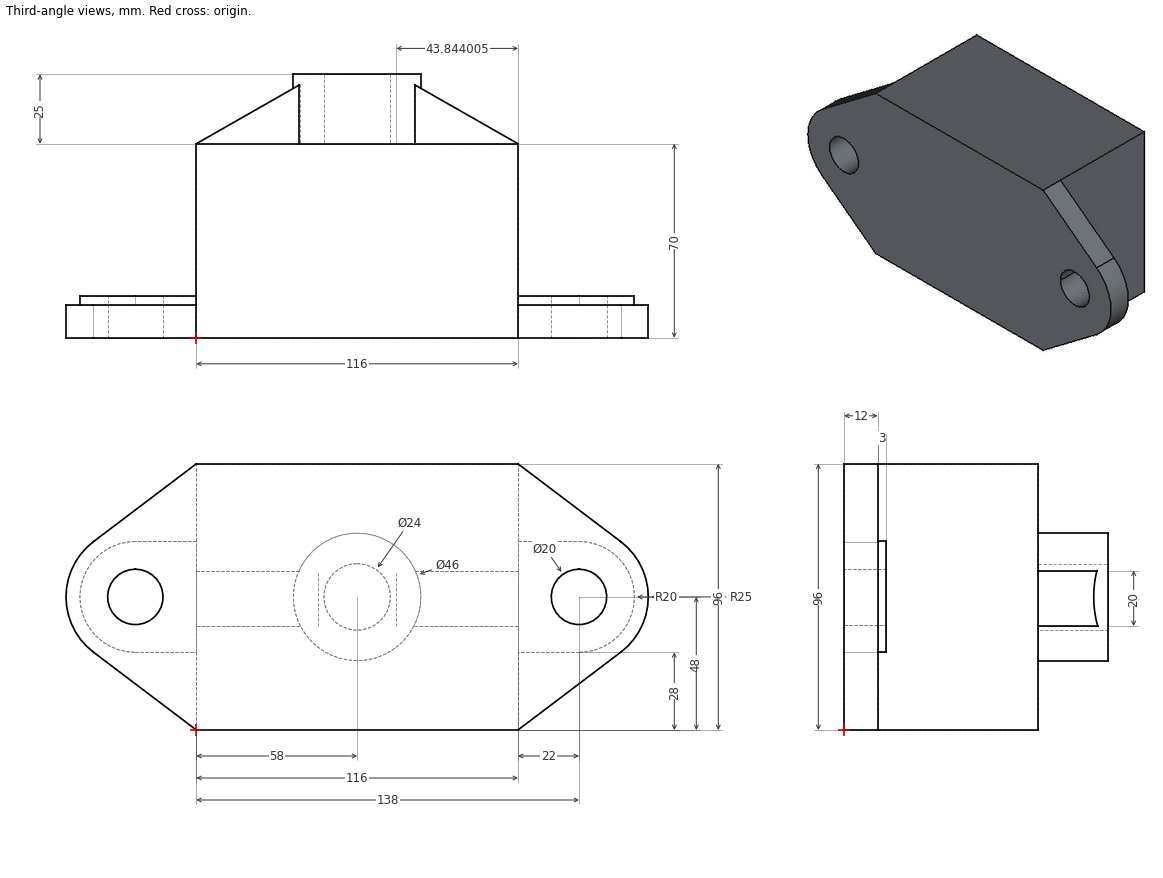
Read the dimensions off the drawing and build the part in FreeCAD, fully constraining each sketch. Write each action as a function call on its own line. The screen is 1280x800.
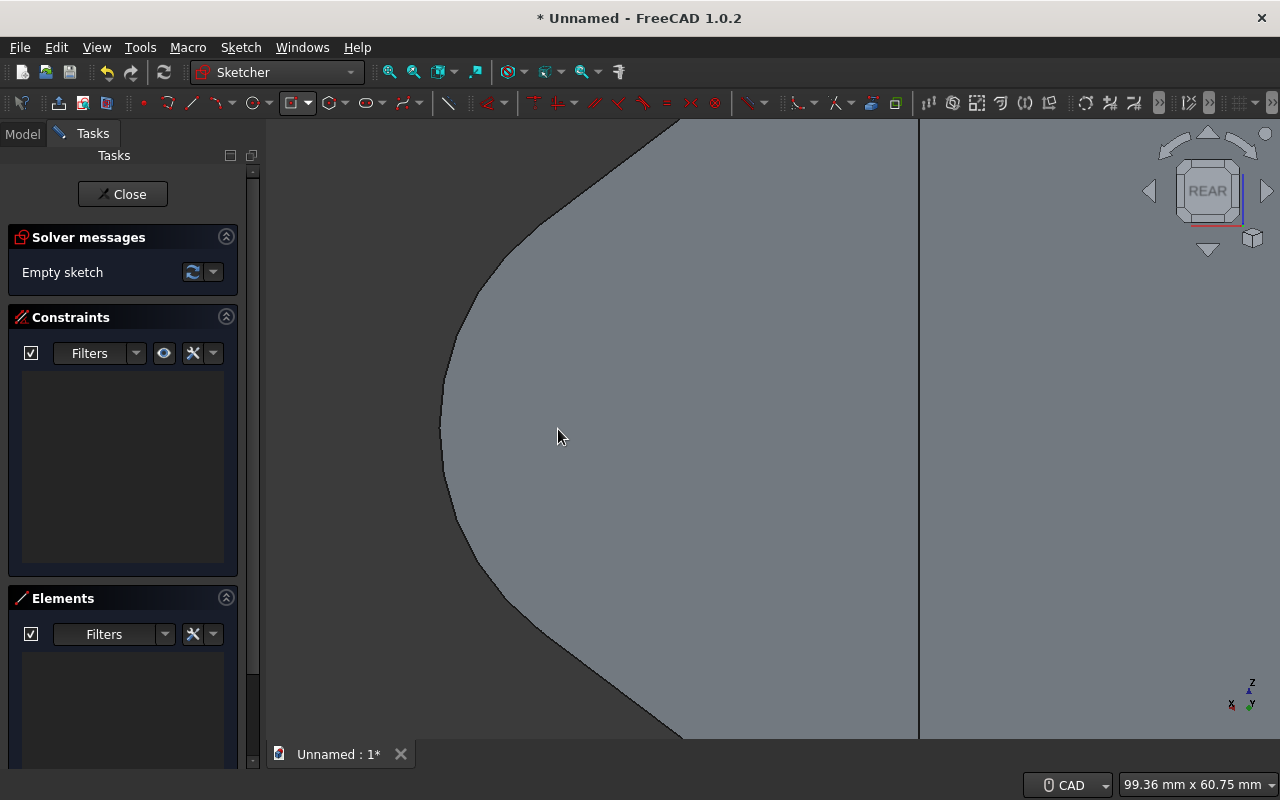
click(168, 104)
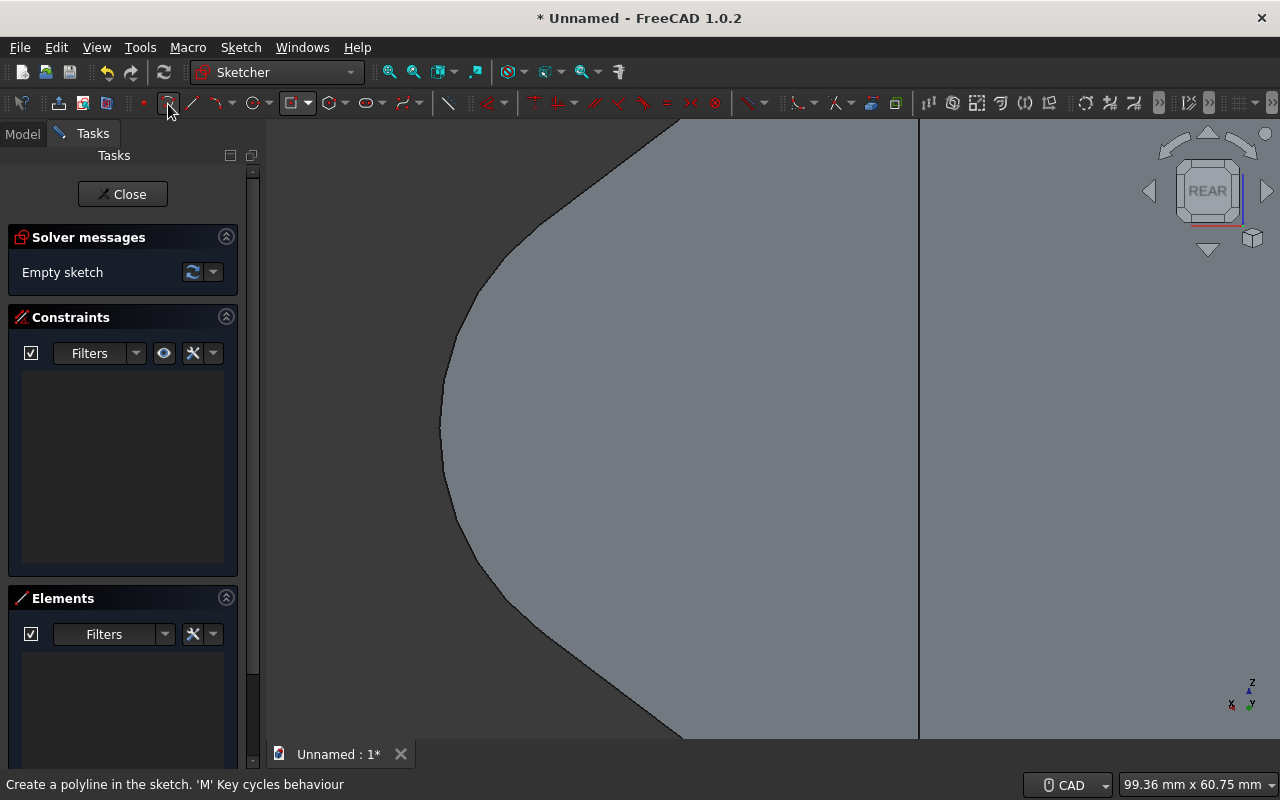
click(695, 632)
click(919, 632)
click(919, 224)
click(695, 224)
right_click(695, 224)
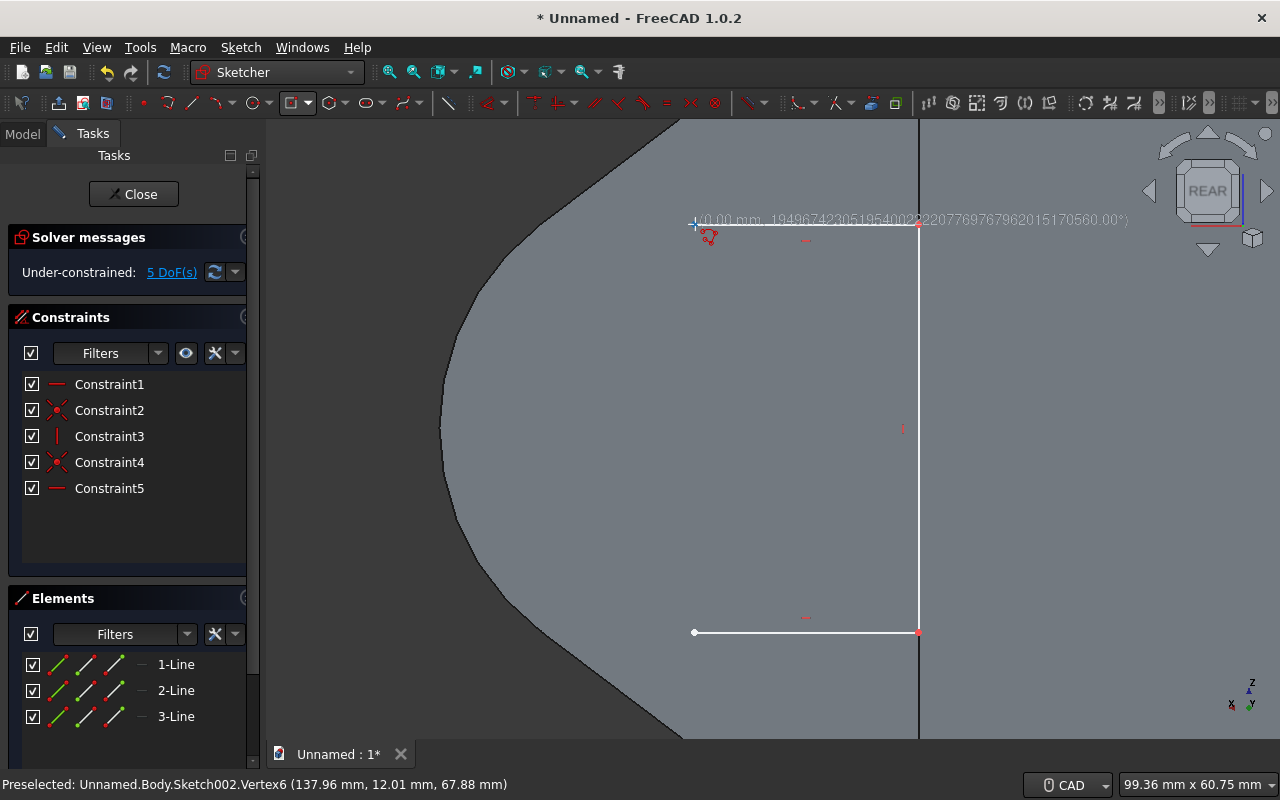
click(216, 104)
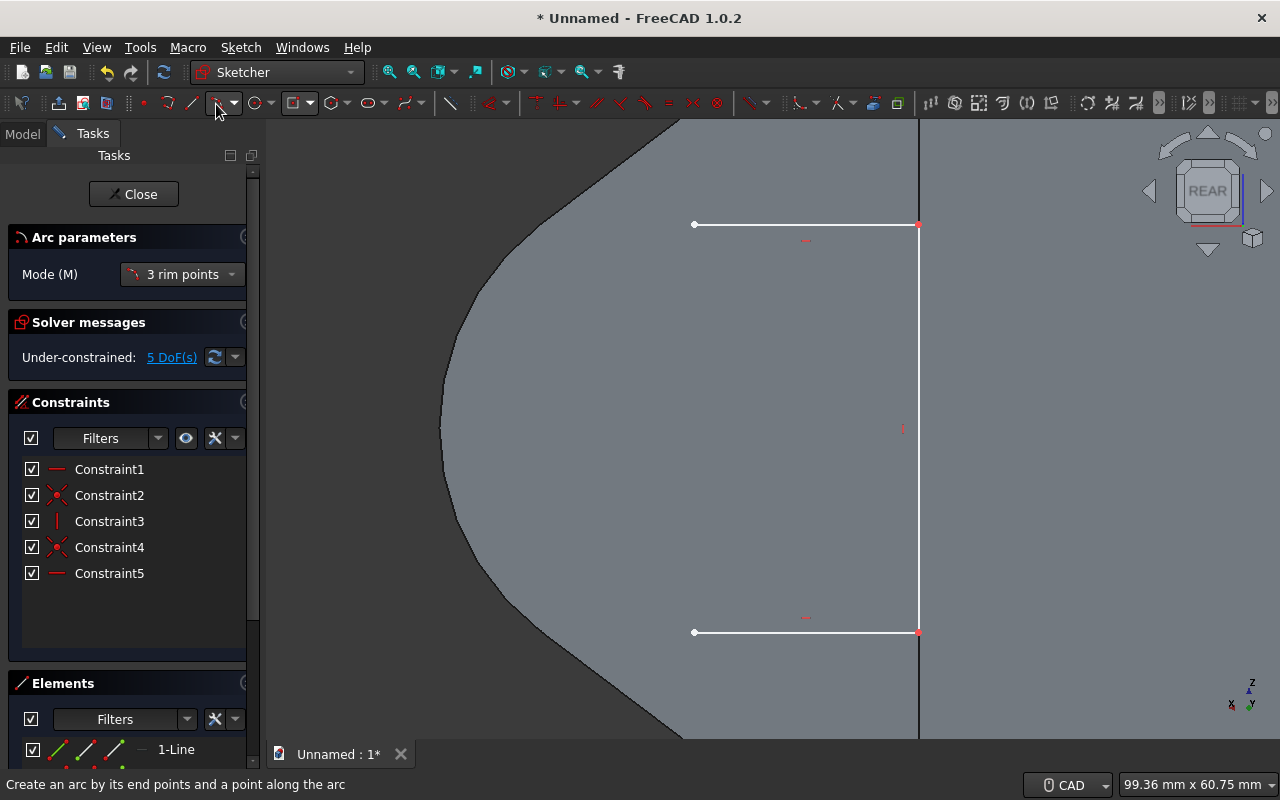
click(695, 225)
click(695, 633)
click(490, 428)
key(Escape)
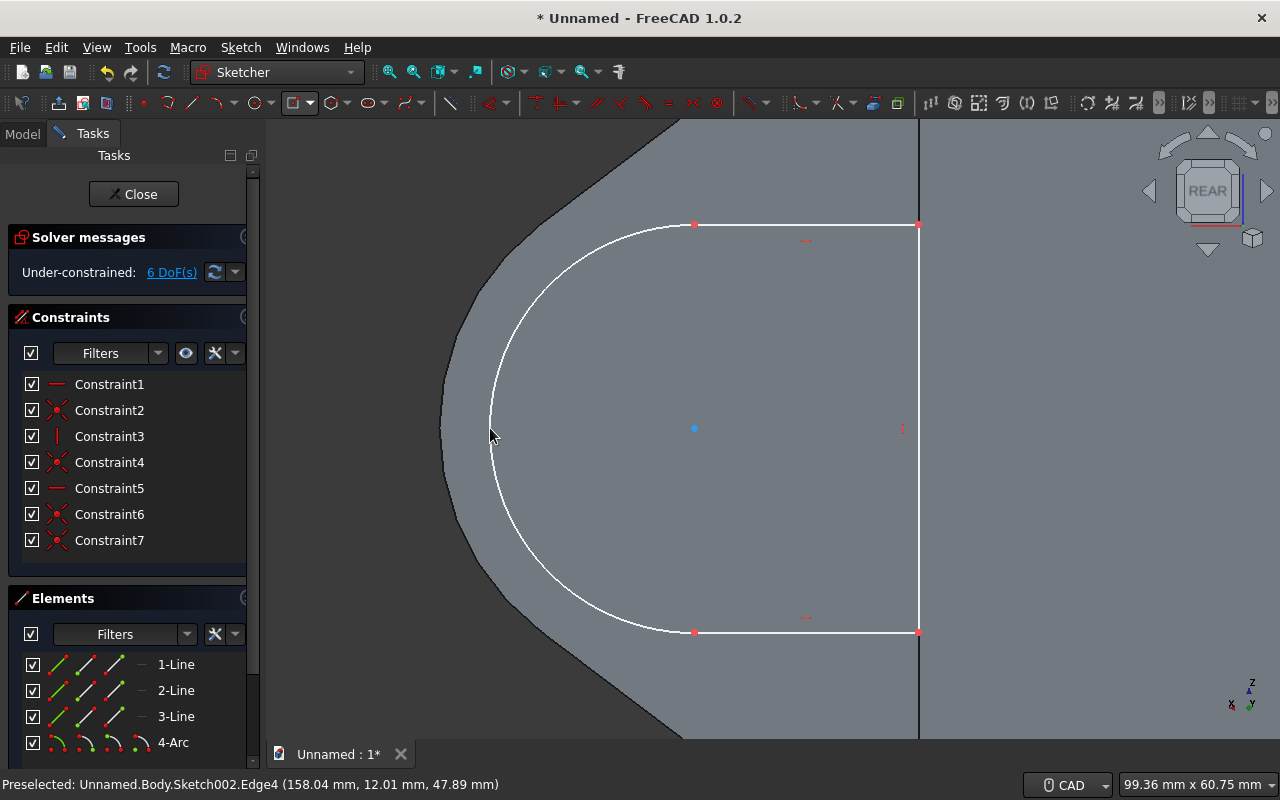
click(762, 633)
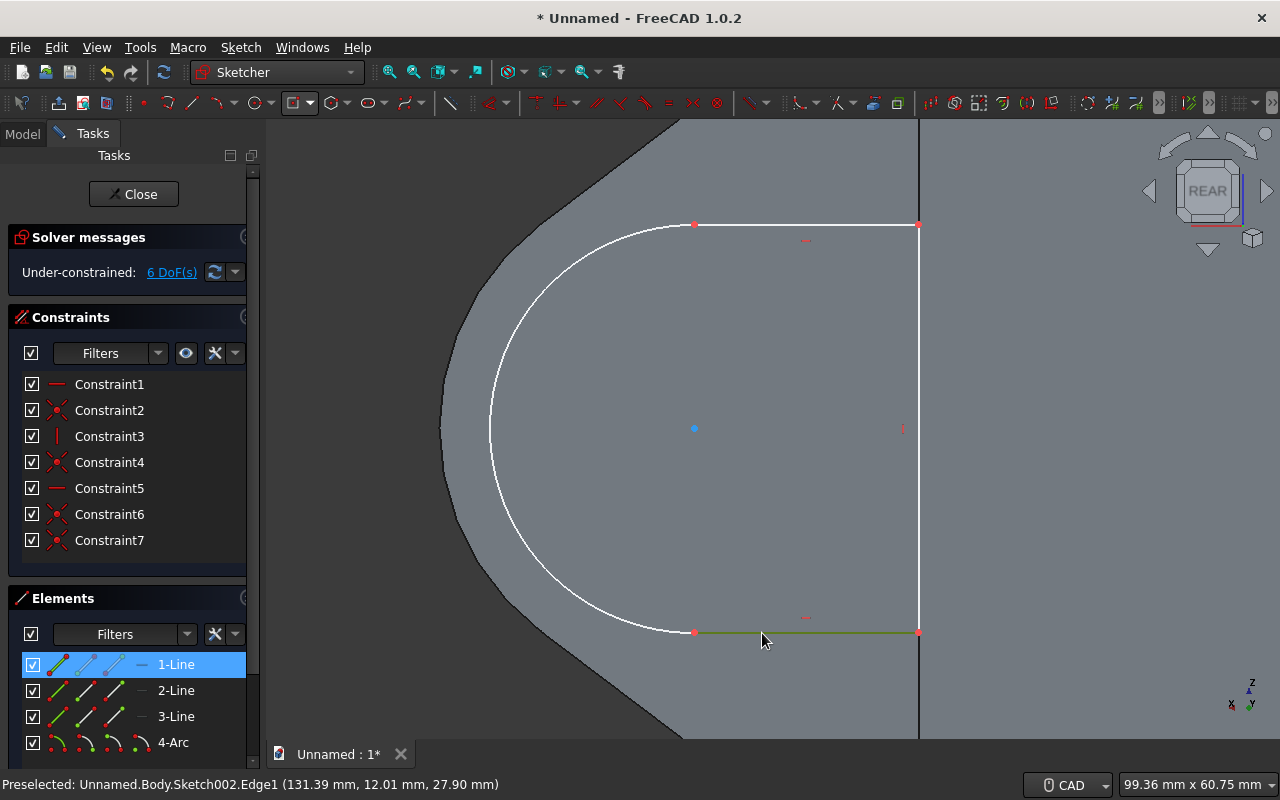
click(529, 309)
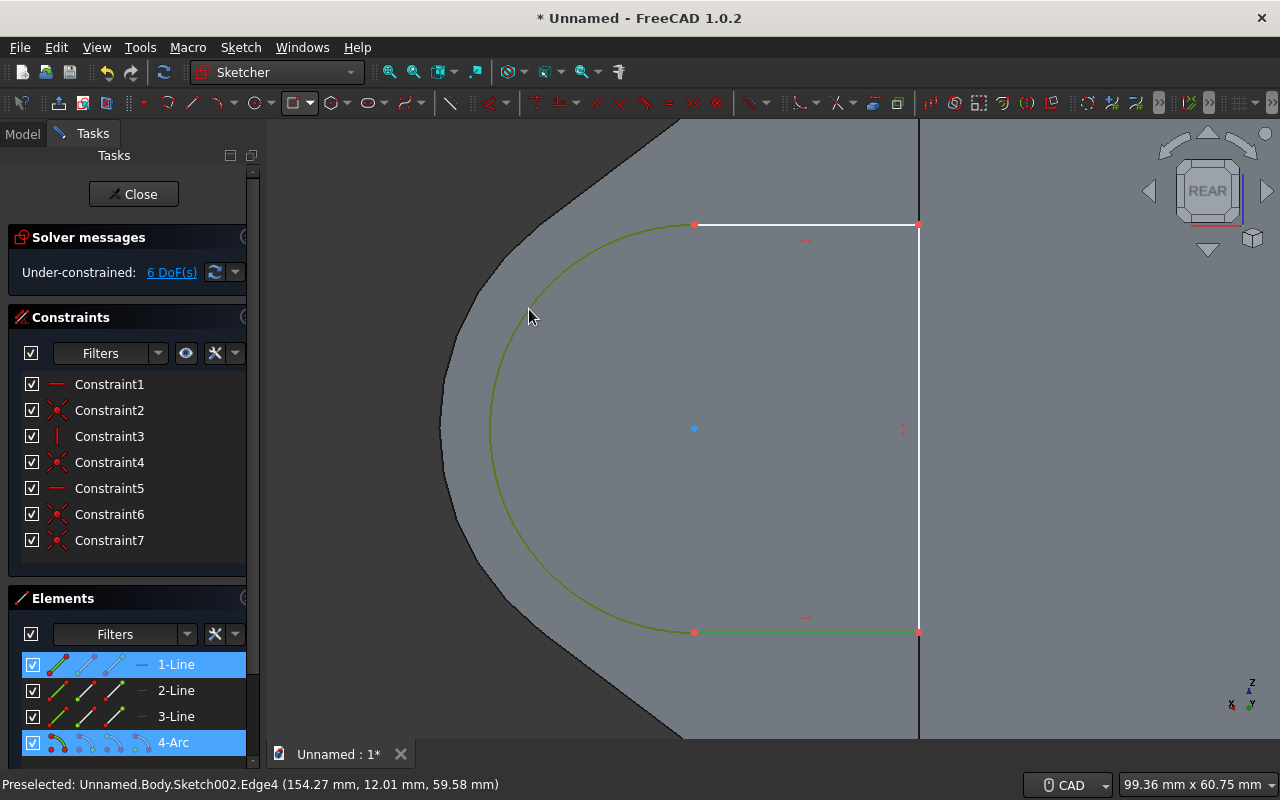
click(646, 104)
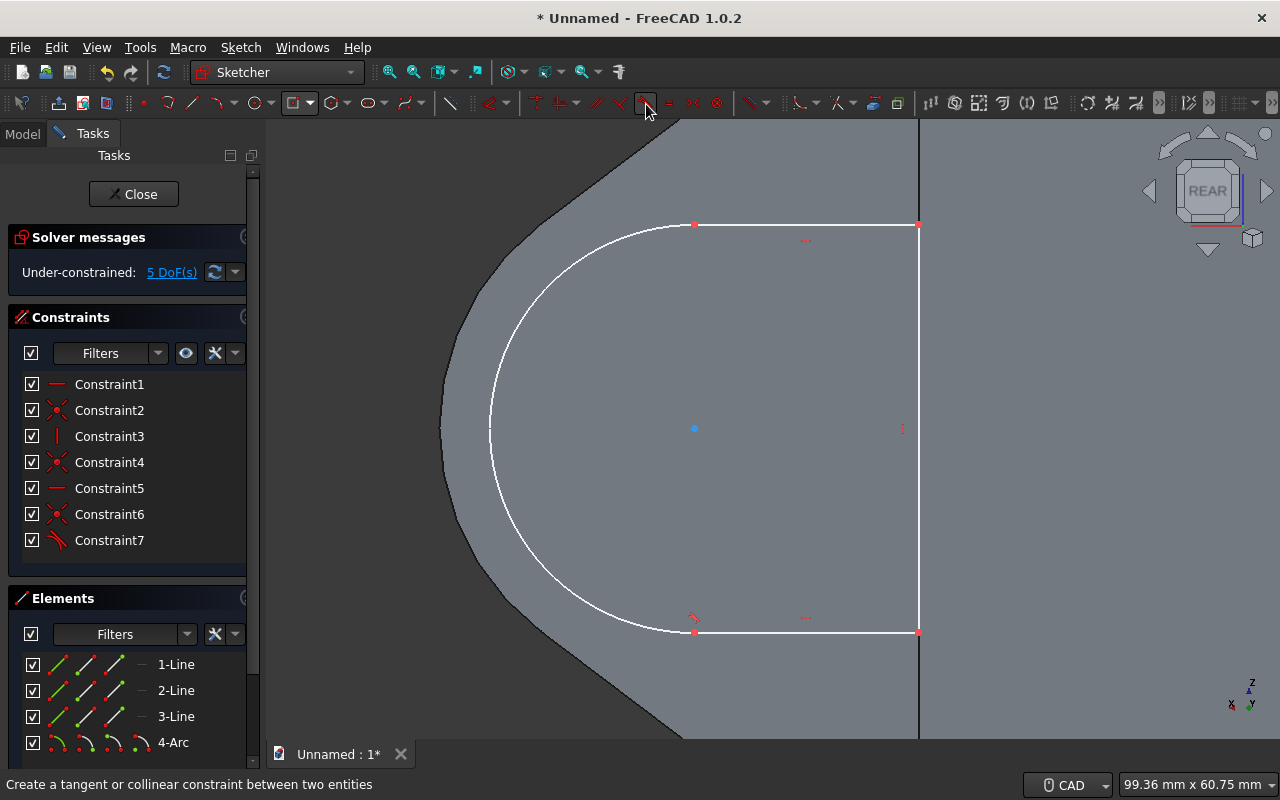
click(852, 225)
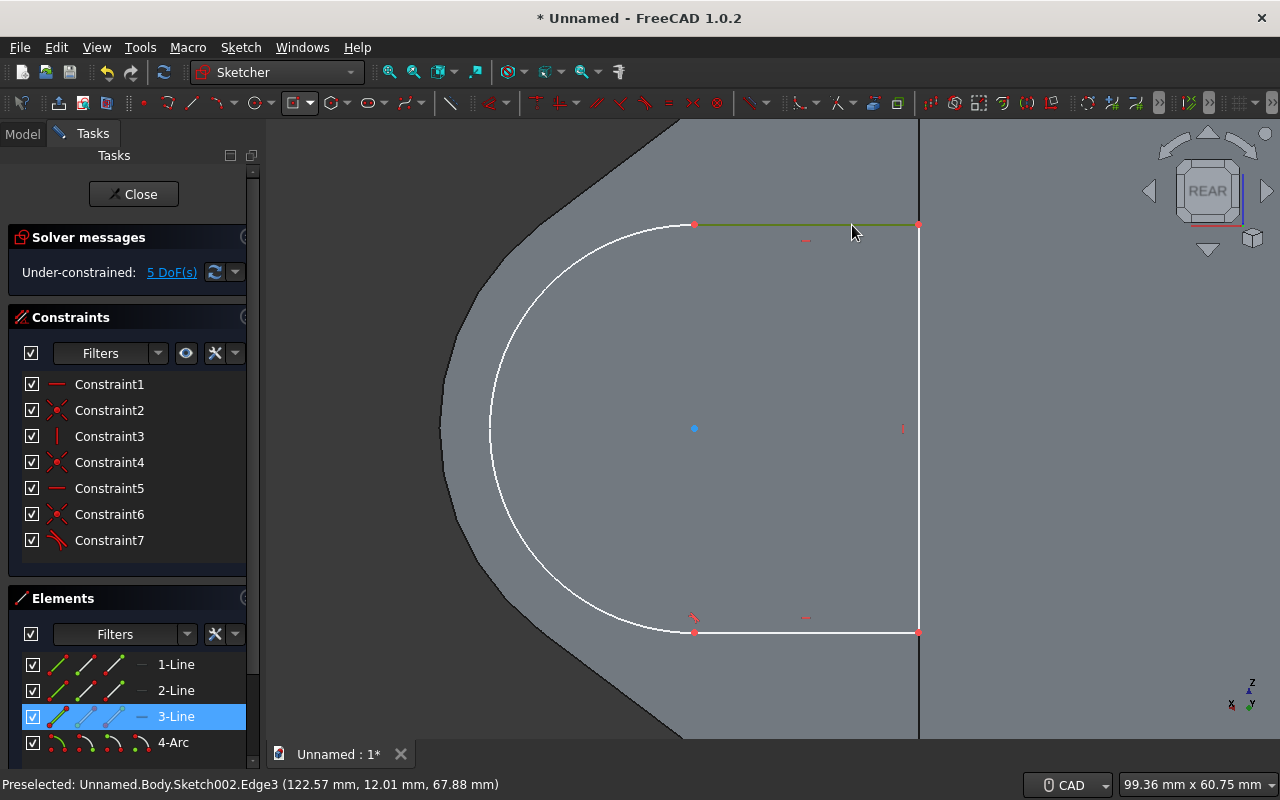
click(529, 309)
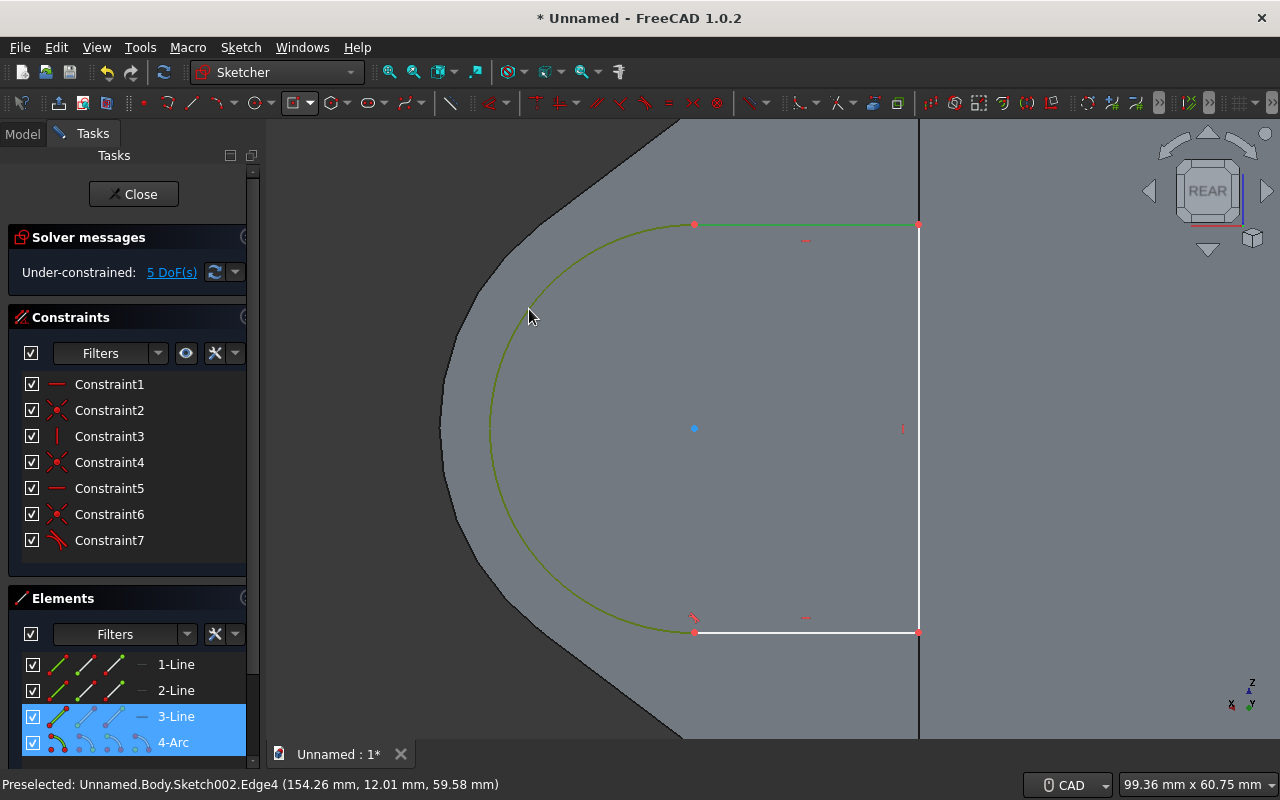
click(646, 104)